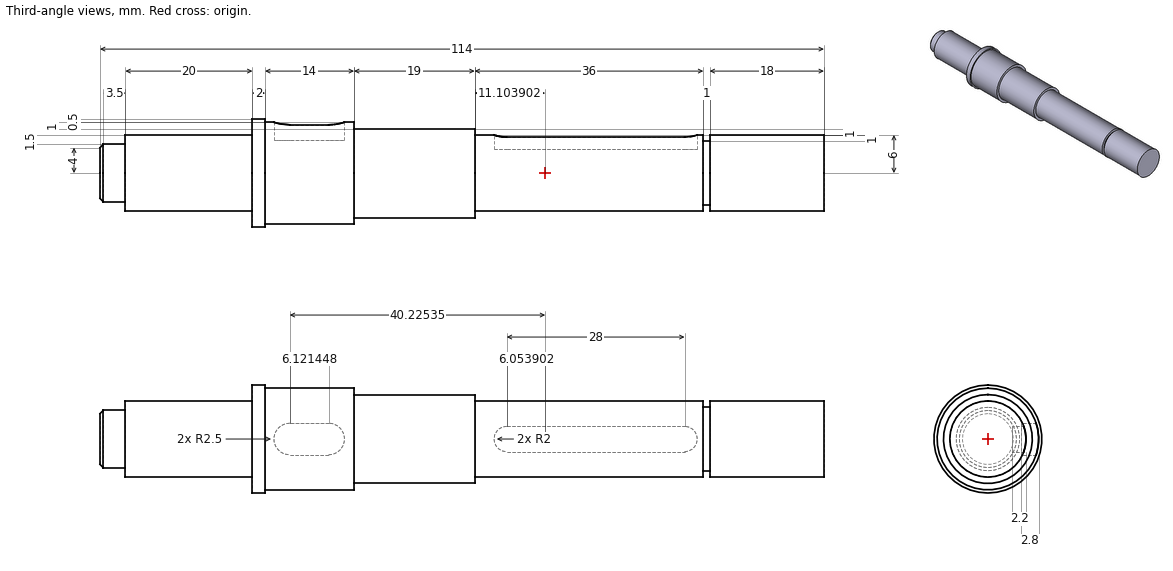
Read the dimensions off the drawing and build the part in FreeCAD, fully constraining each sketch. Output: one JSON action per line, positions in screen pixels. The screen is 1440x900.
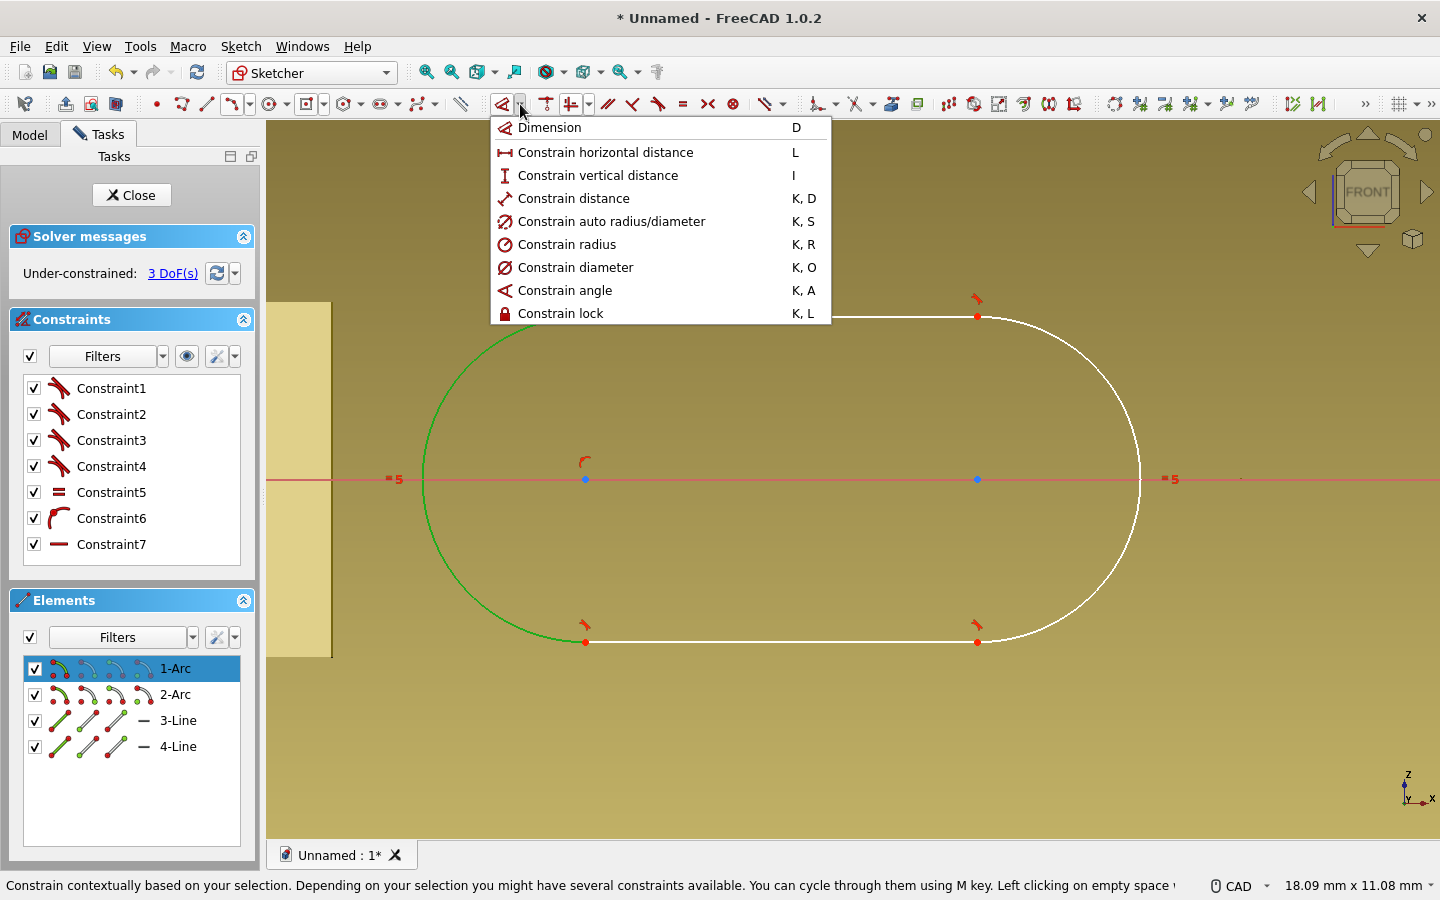
{"action": "left_click", "coordinate": [661, 244]}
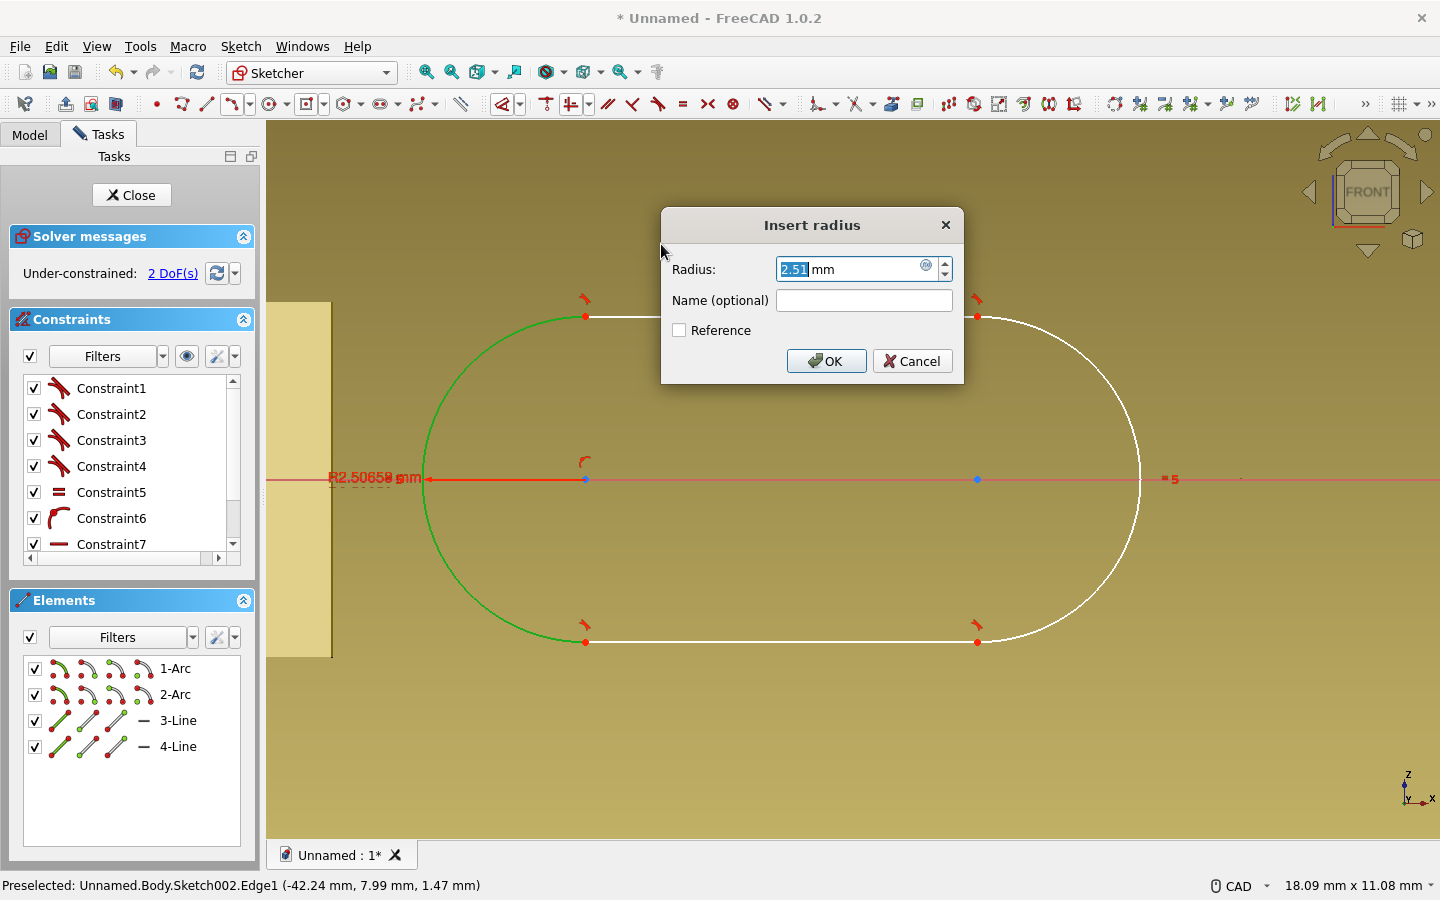
{"action": "type", "text": "2.5"}
{"action": "key", "text": "Return"}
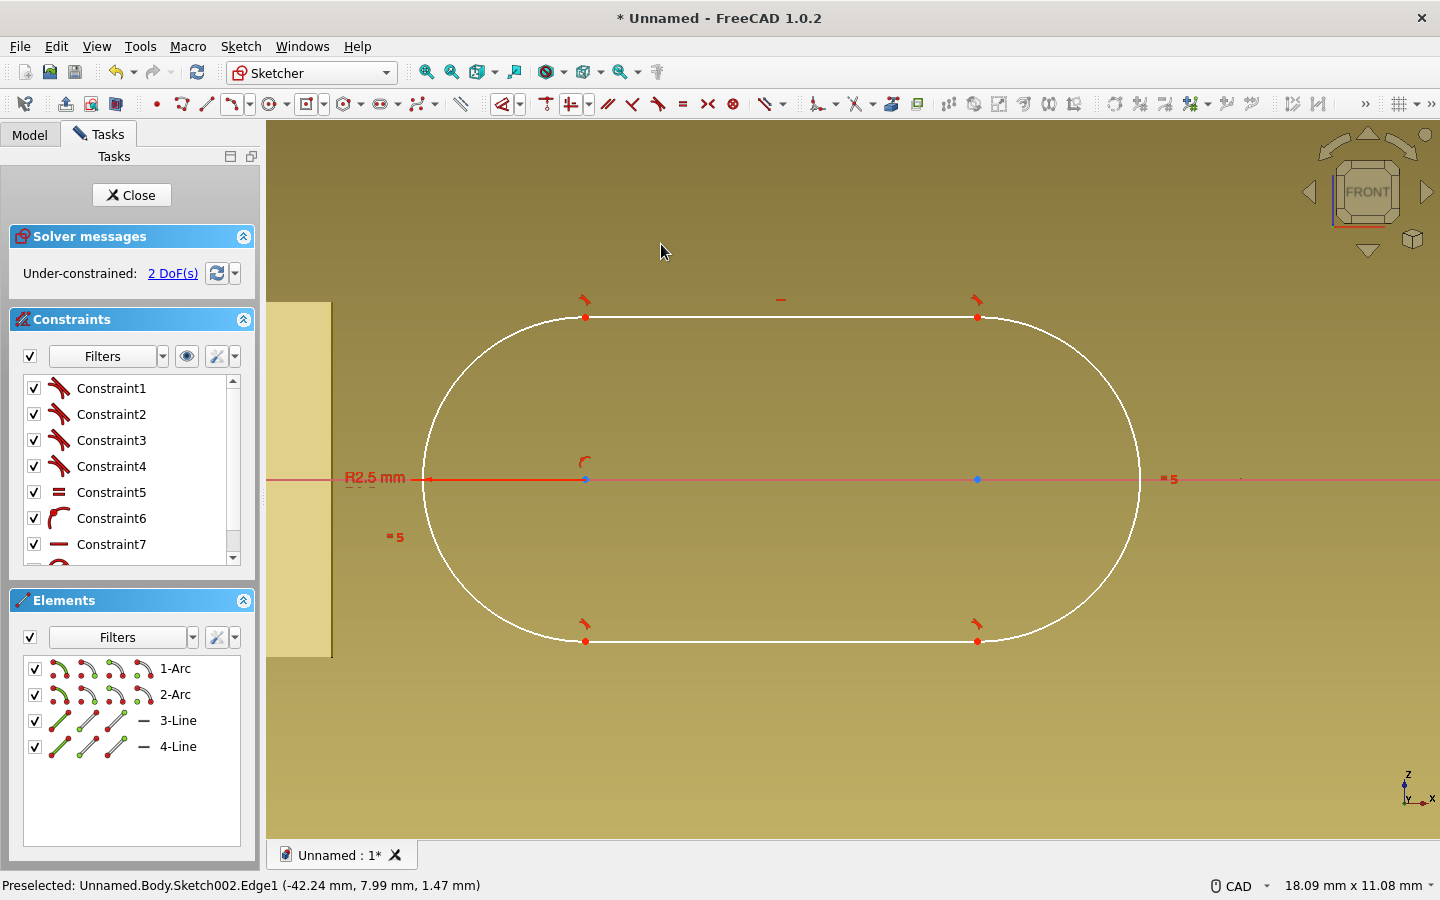
{"action": "left_click", "coordinate": [703, 317]}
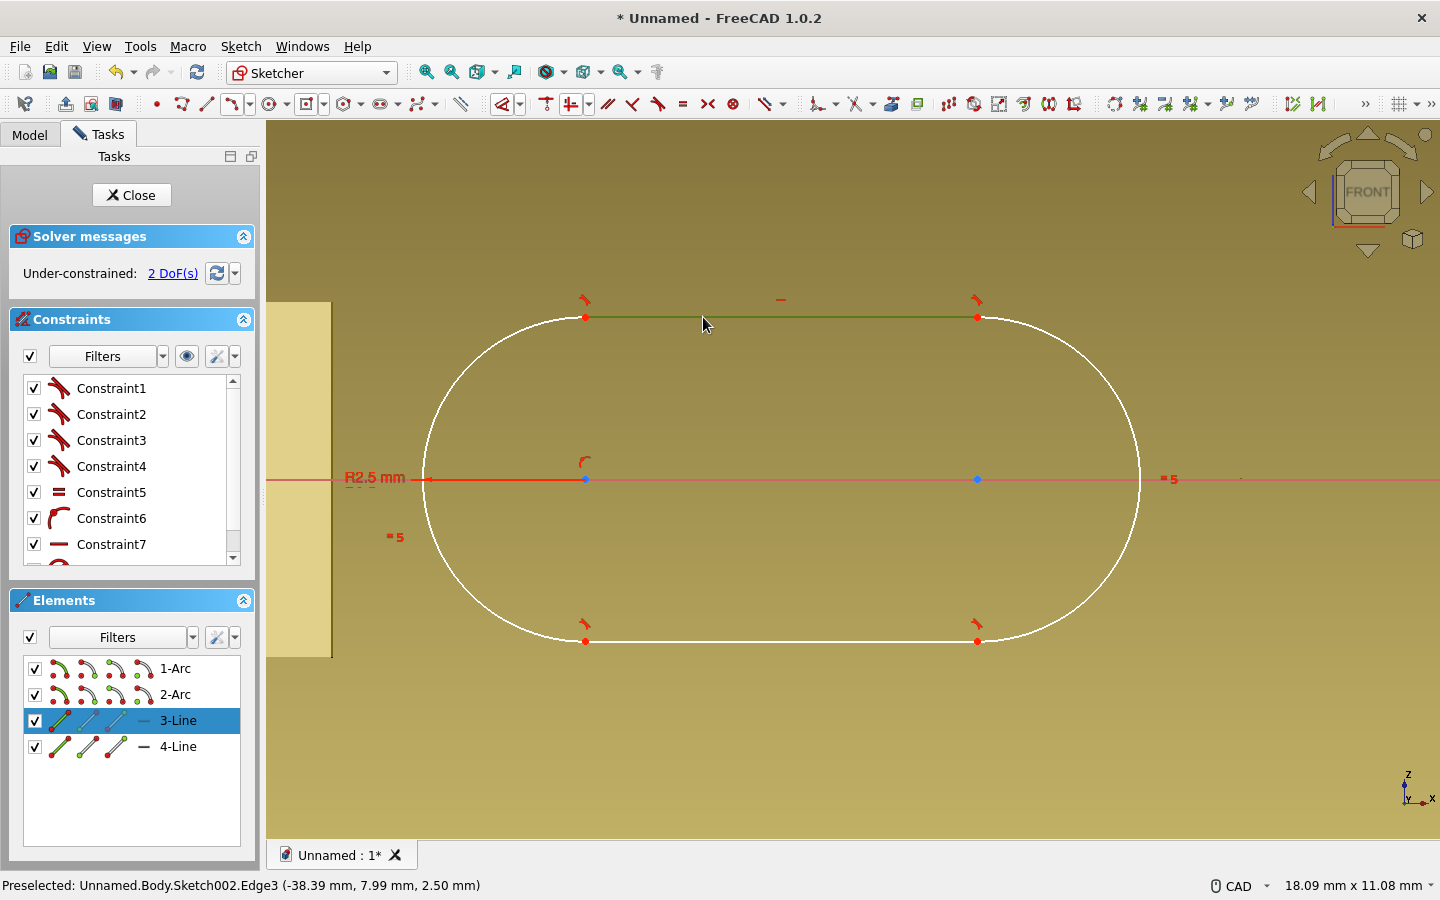
{"action": "key", "text": "l"}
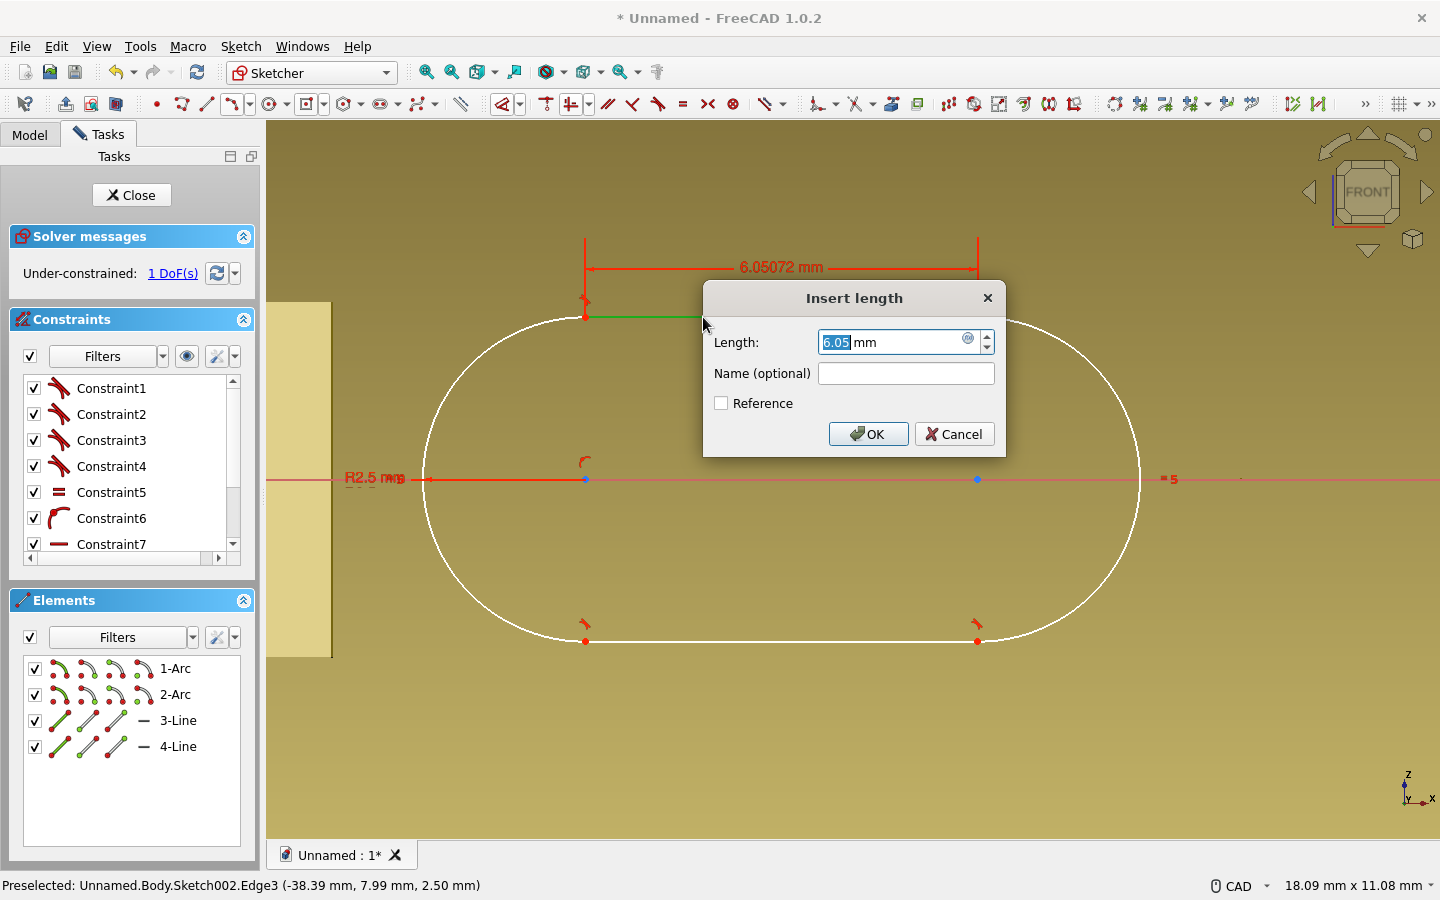
{"action": "type", "text": "6.121448"}
{"action": "key", "text": "Return"}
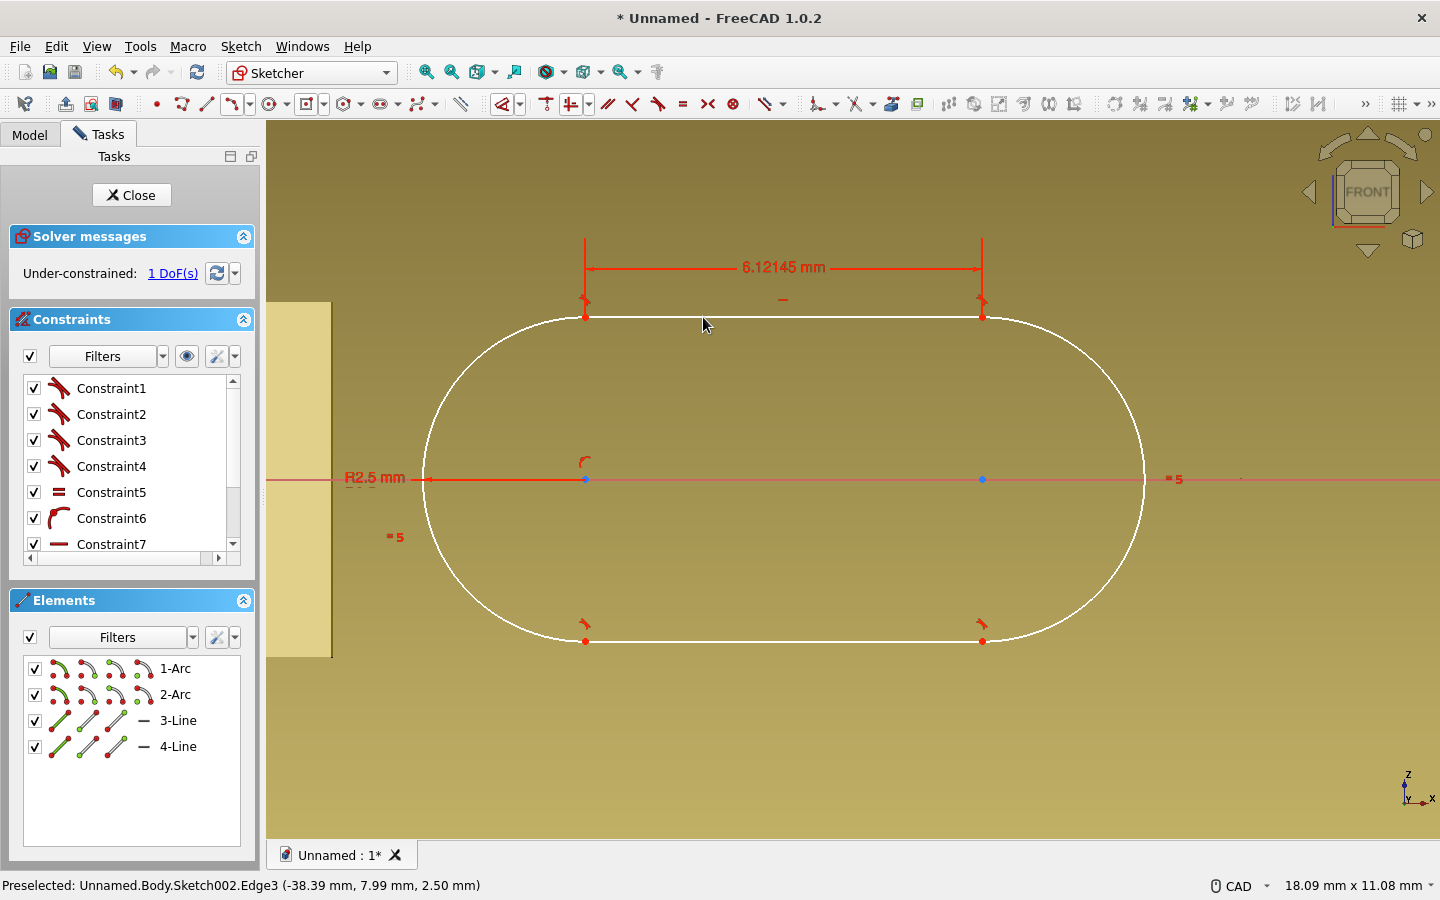
{"action": "left_click", "coordinate": [585, 317]}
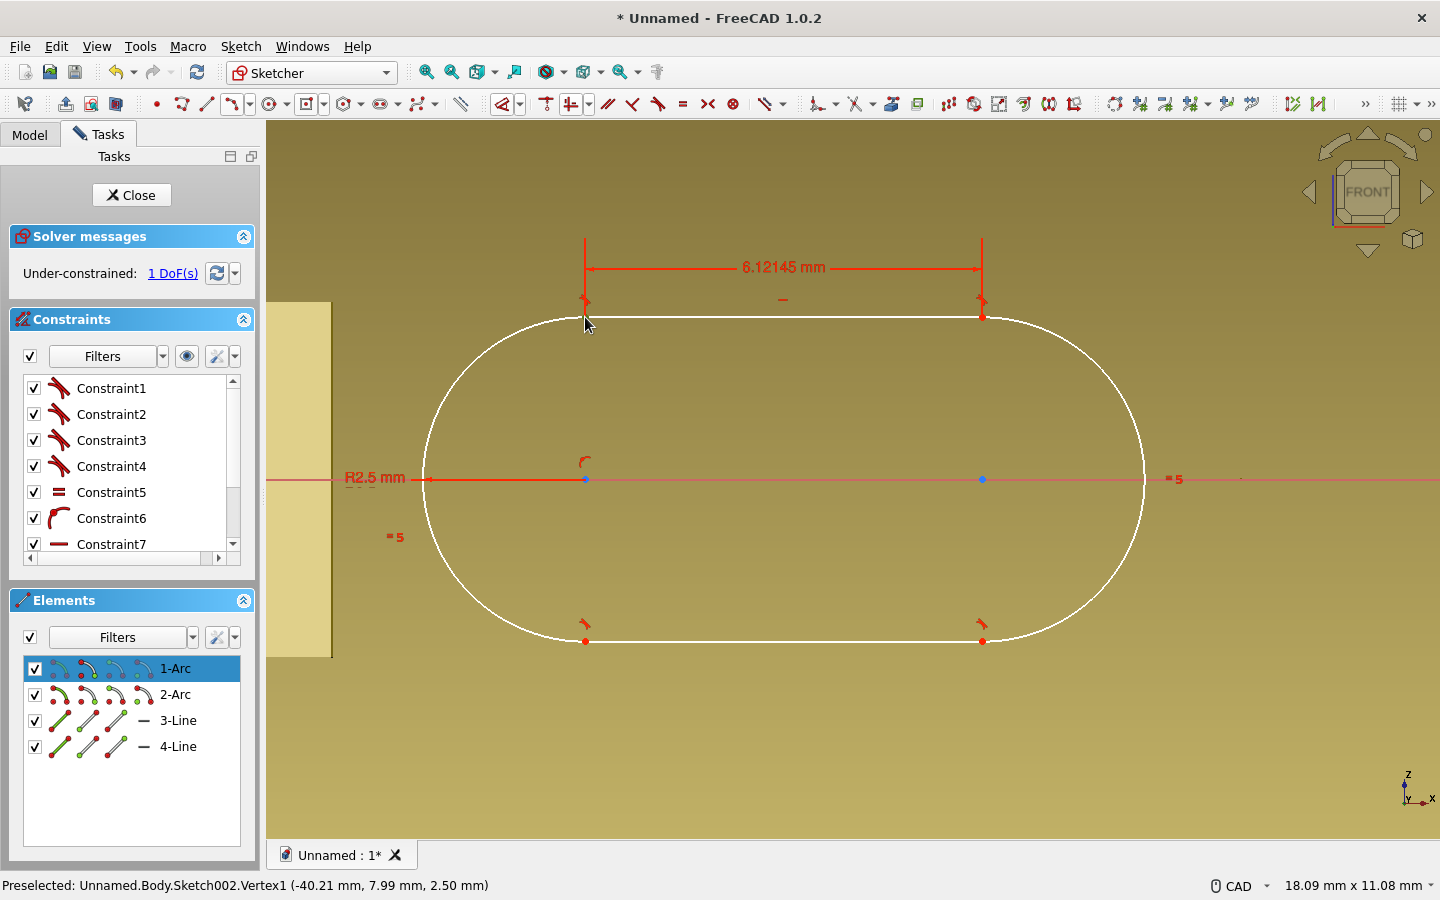
{"action": "key", "text": "l"}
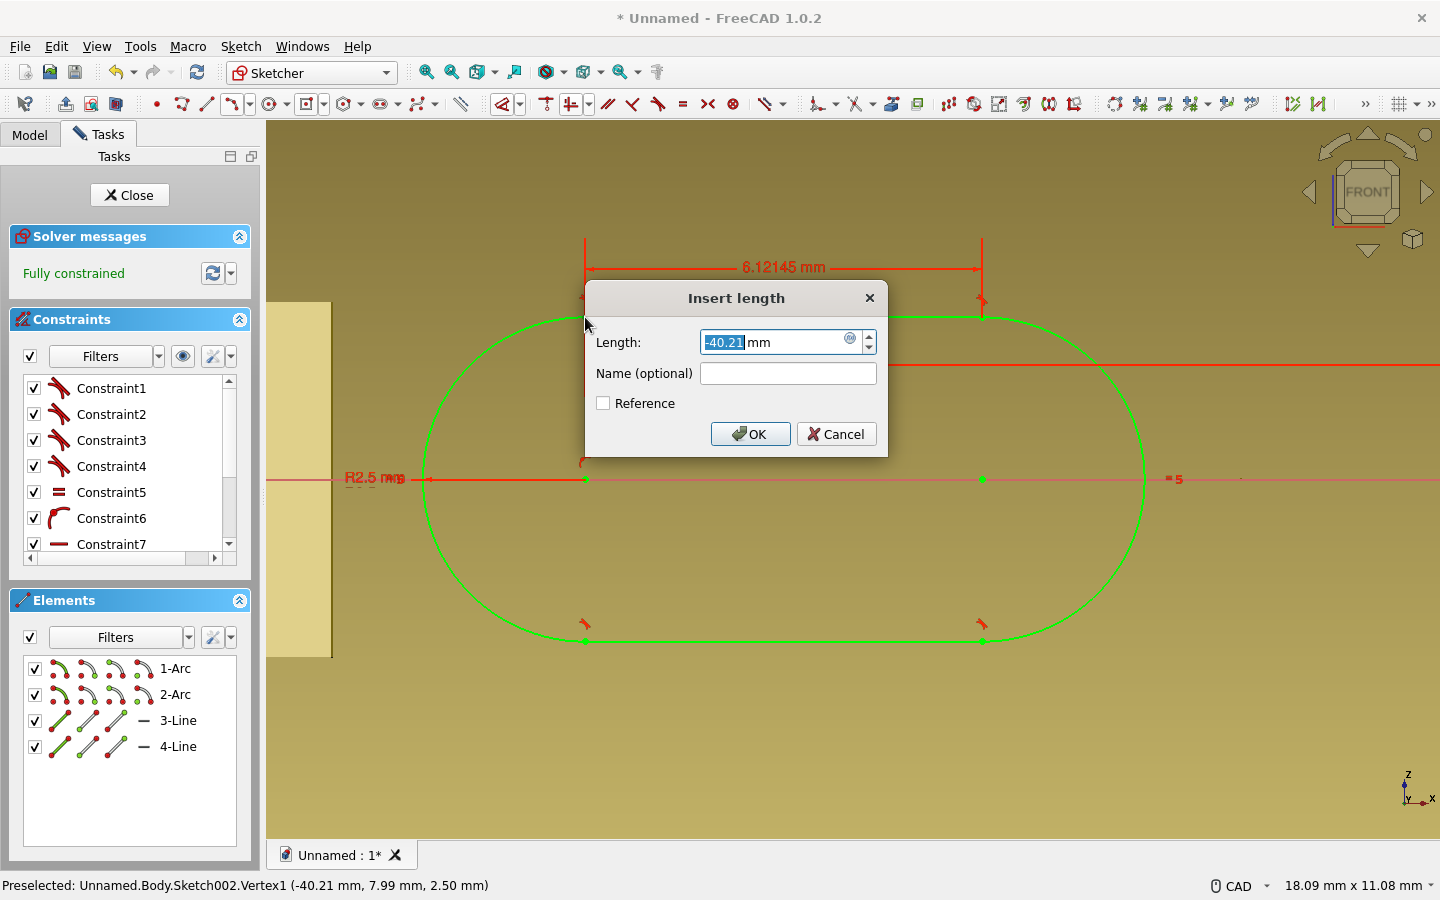
{"action": "type", "text": "-40.22535"}
{"action": "key", "text": "Return"}